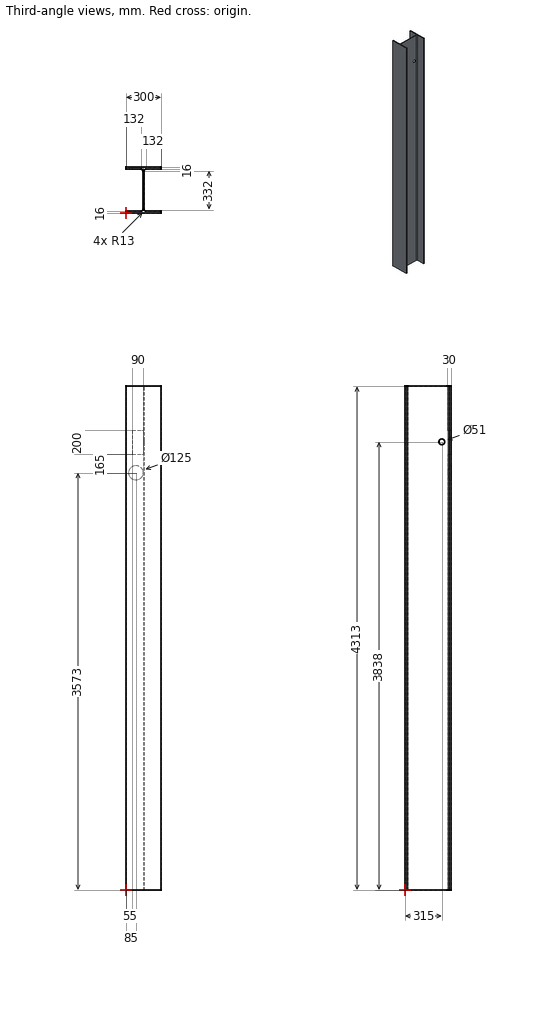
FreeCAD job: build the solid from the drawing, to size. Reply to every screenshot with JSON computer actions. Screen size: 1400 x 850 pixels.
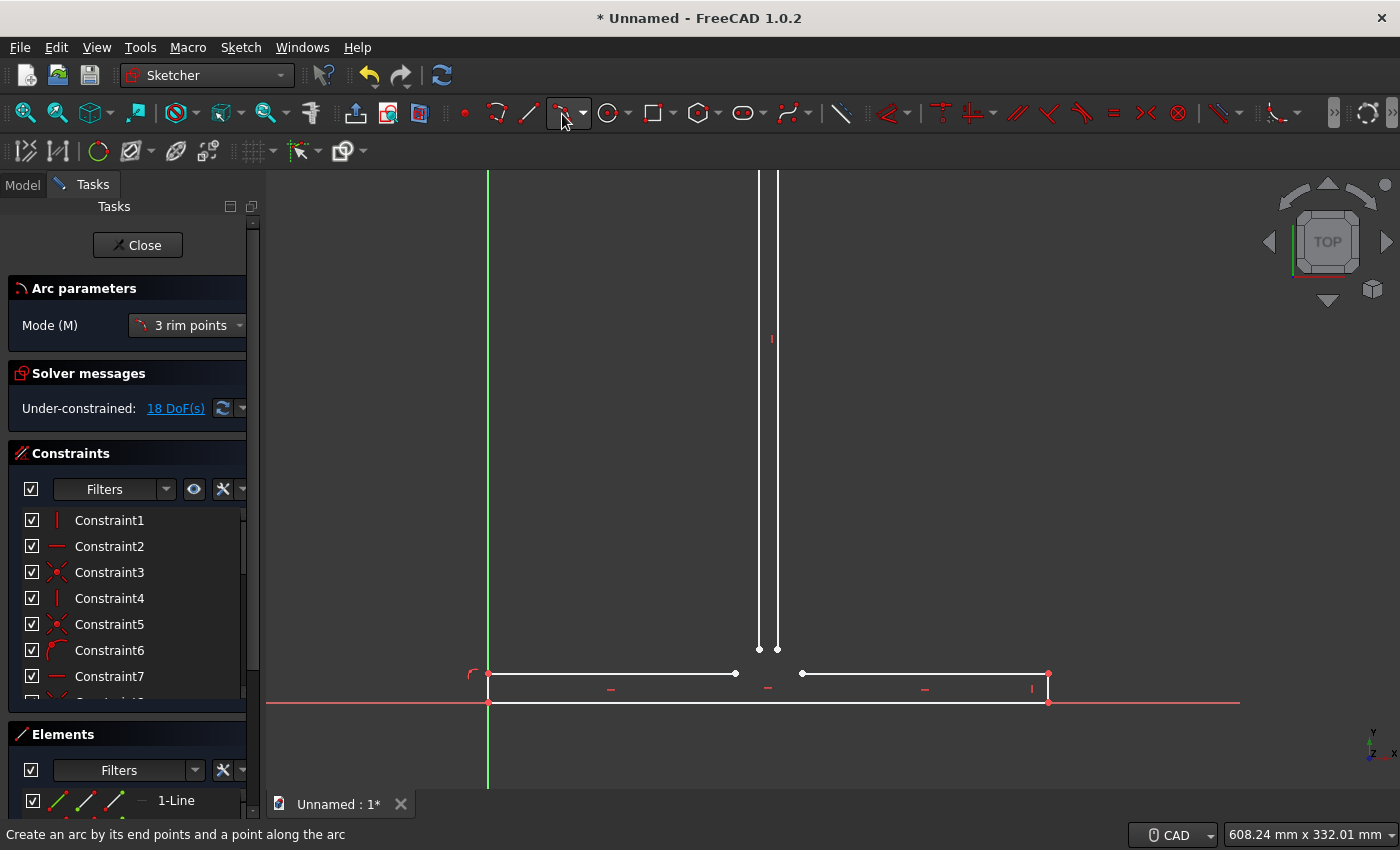
{"action": "scroll", "coordinate": [760, 650], "scroll_direction": "down", "scroll_amount": 3}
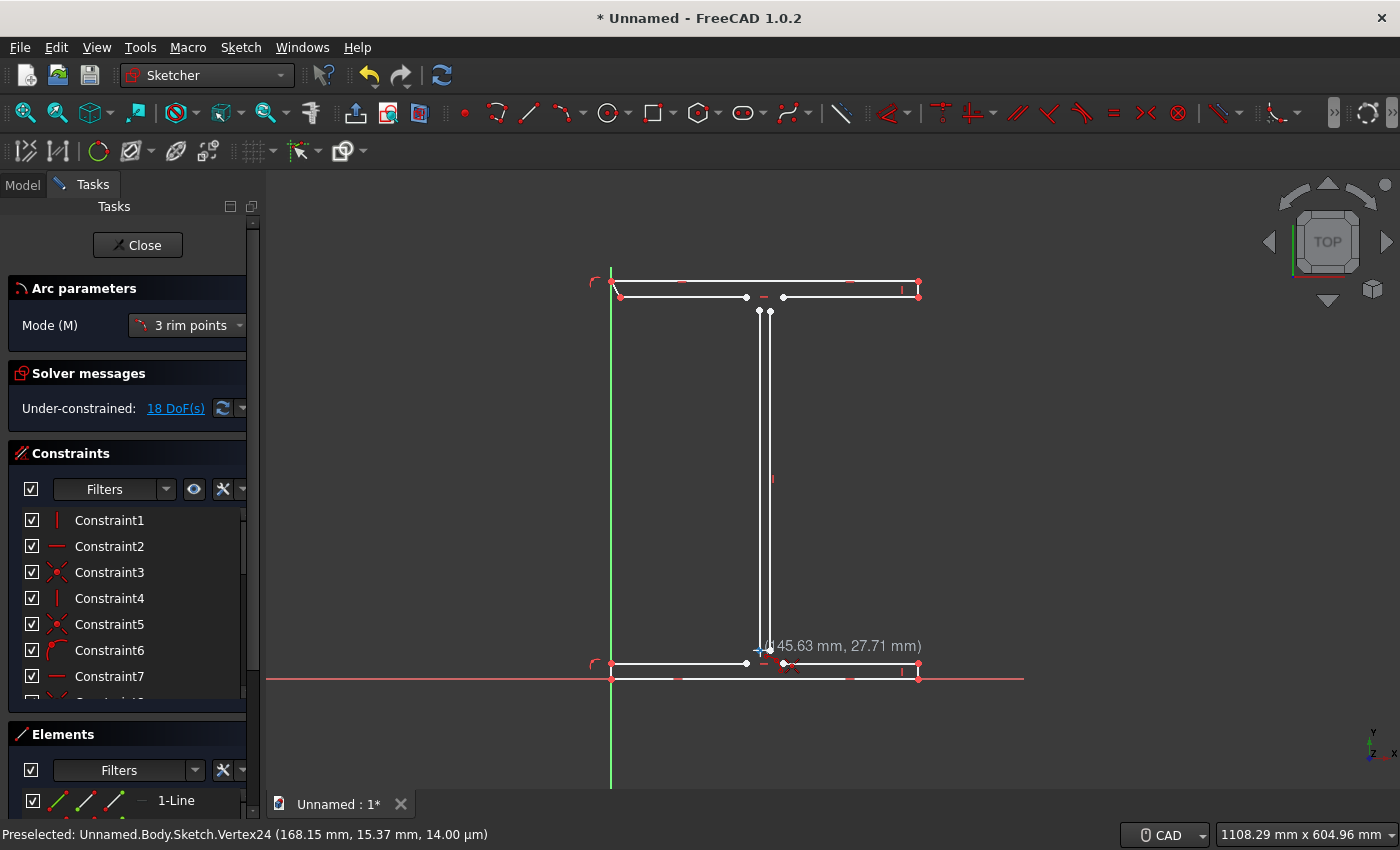
{"action": "scroll", "coordinate": [770, 310], "scroll_direction": "up", "scroll_amount": 3}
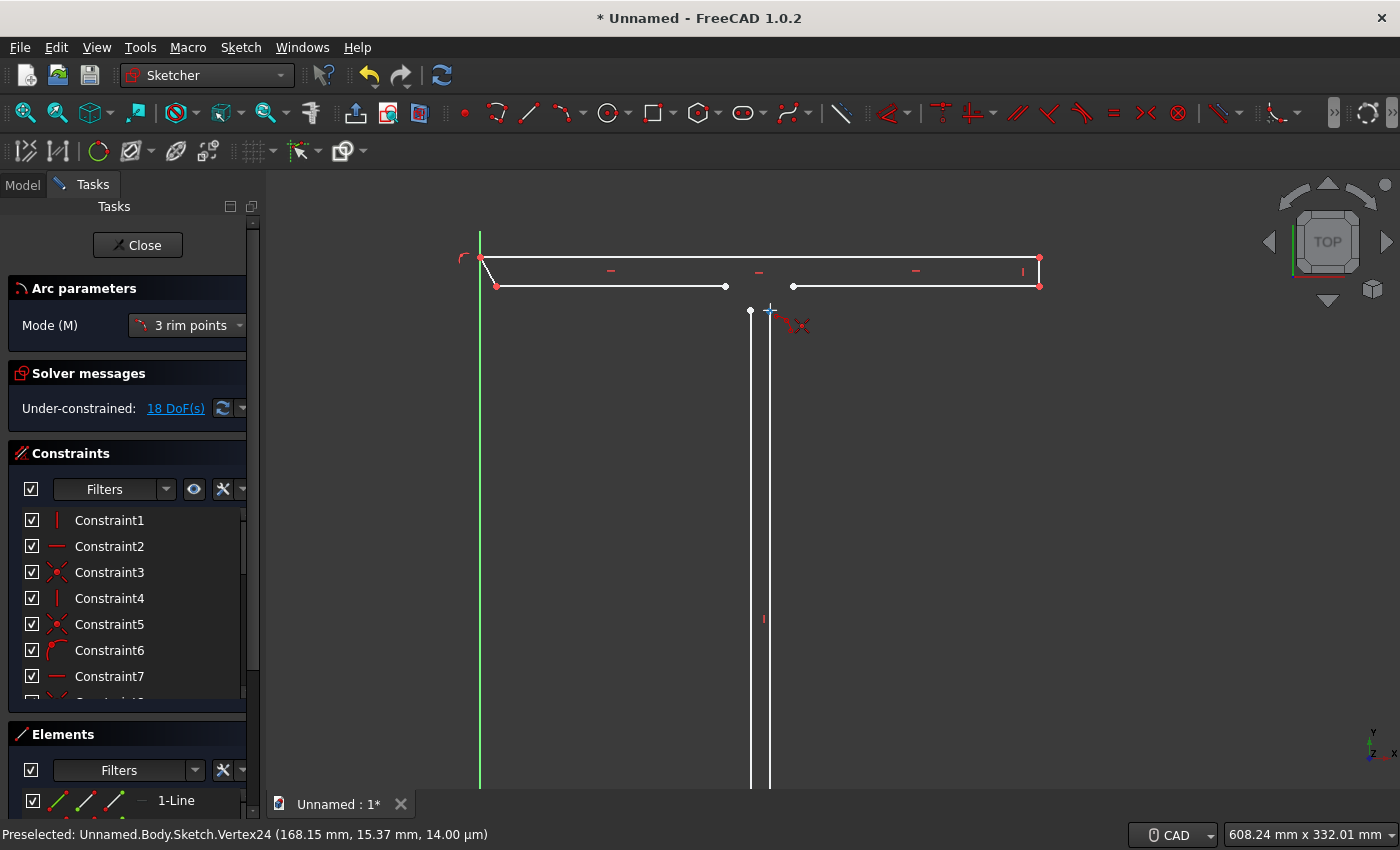
{"action": "left_click", "coordinate": [770, 312]}
{"action": "left_click", "coordinate": [793, 286]}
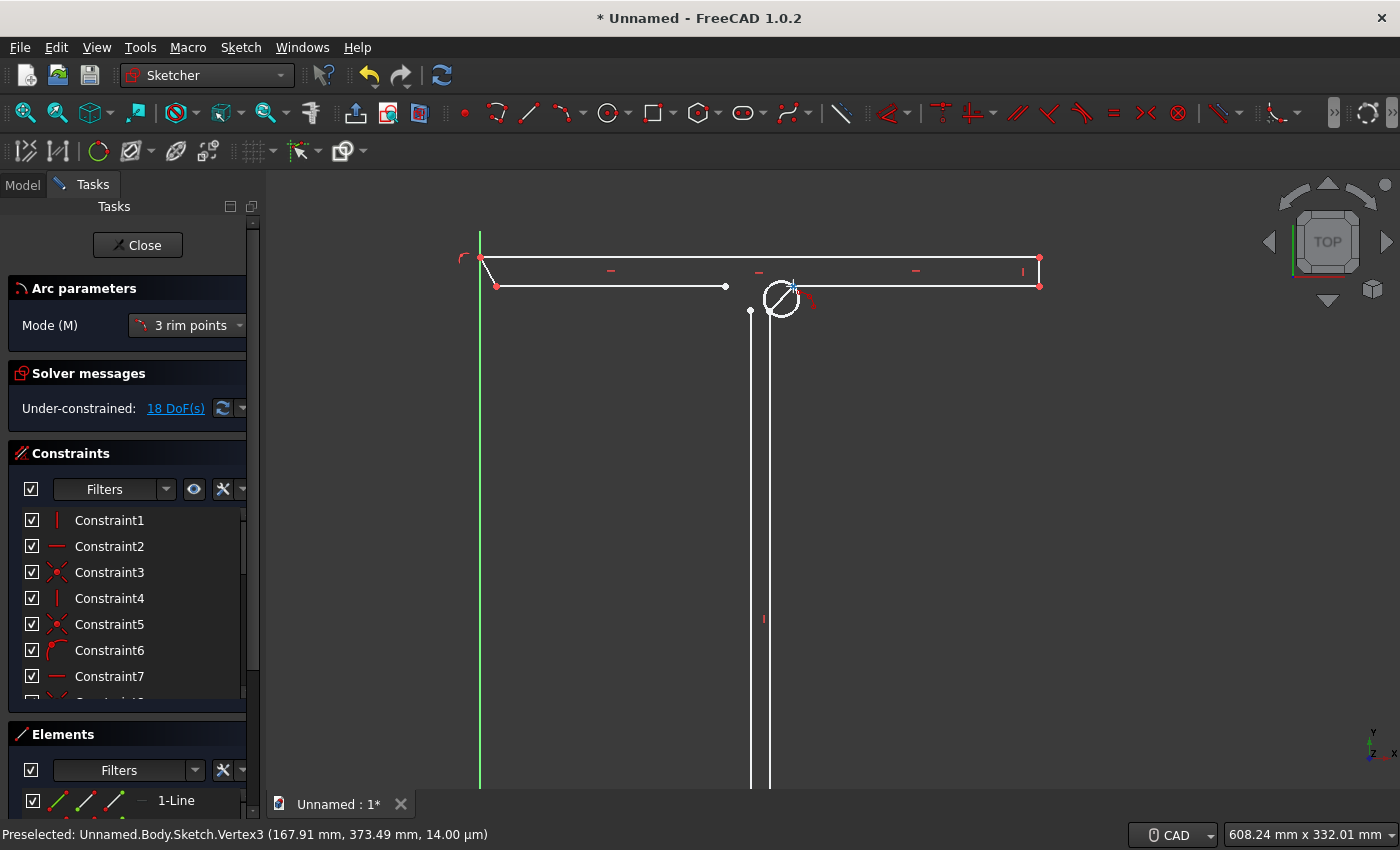
{"action": "scroll", "coordinate": [776, 292], "scroll_direction": "up", "scroll_amount": 5}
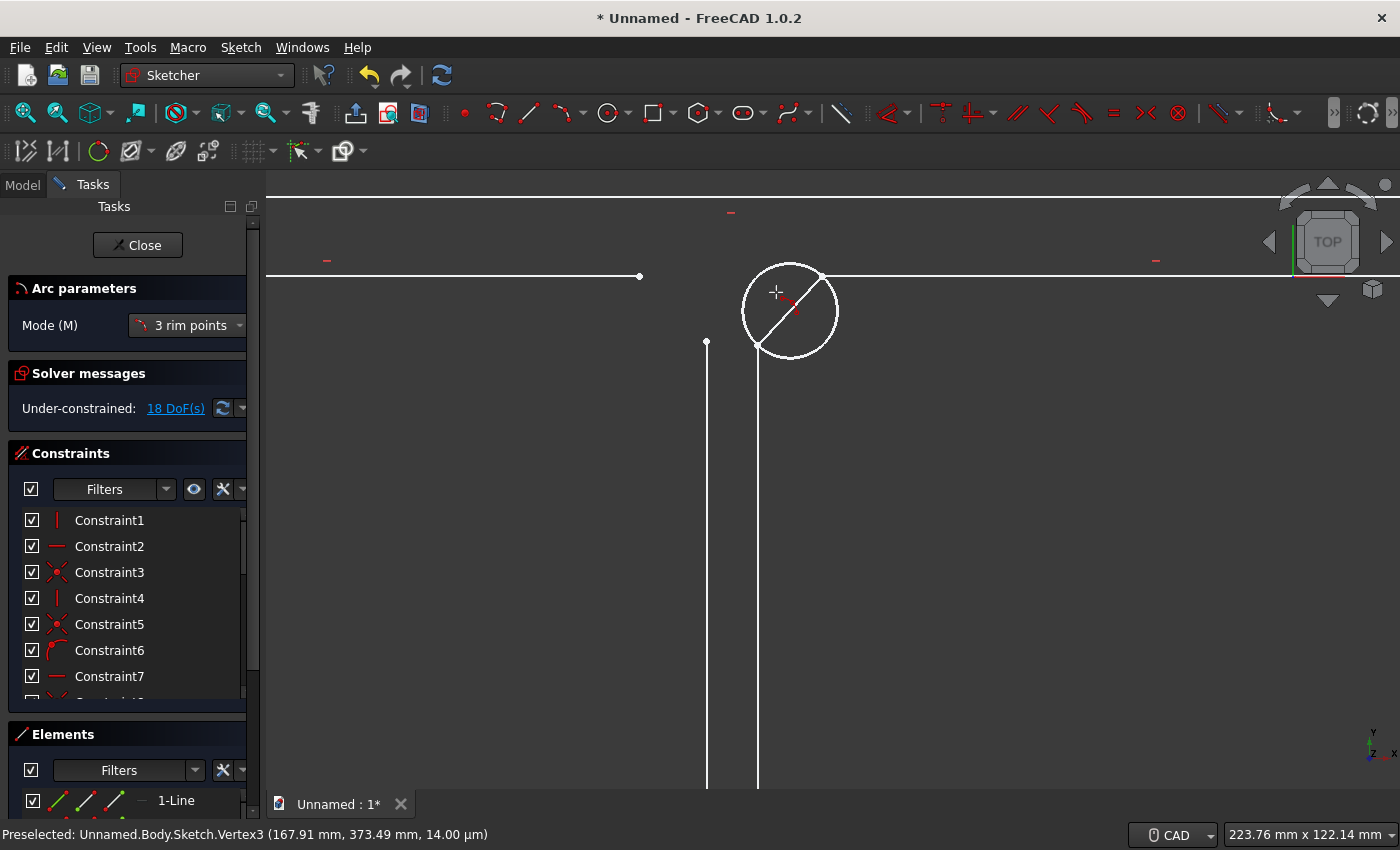
{"action": "left_click", "coordinate": [776, 293]}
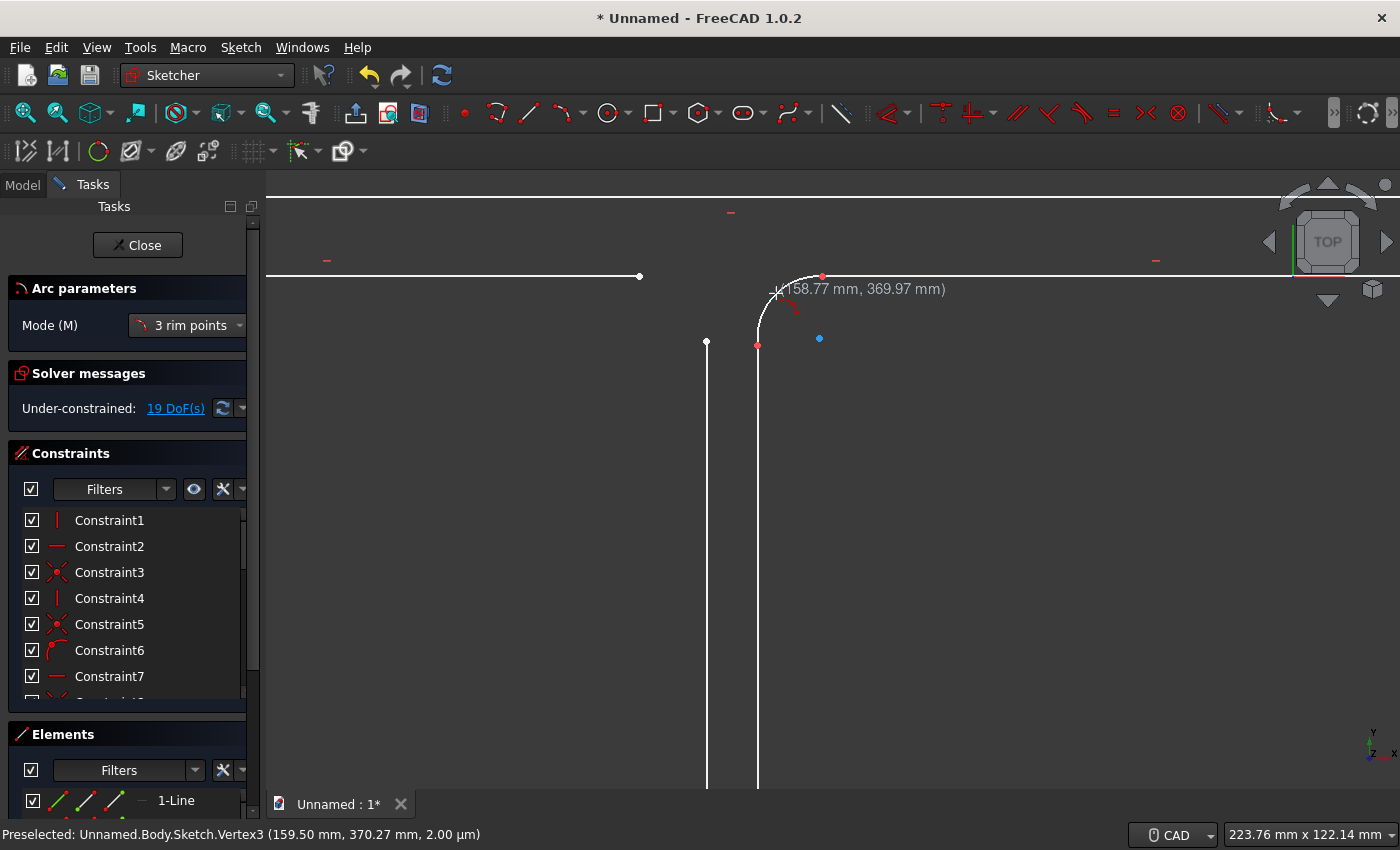
{"action": "scroll", "coordinate": [773, 302], "scroll_direction": "down", "scroll_amount": 8}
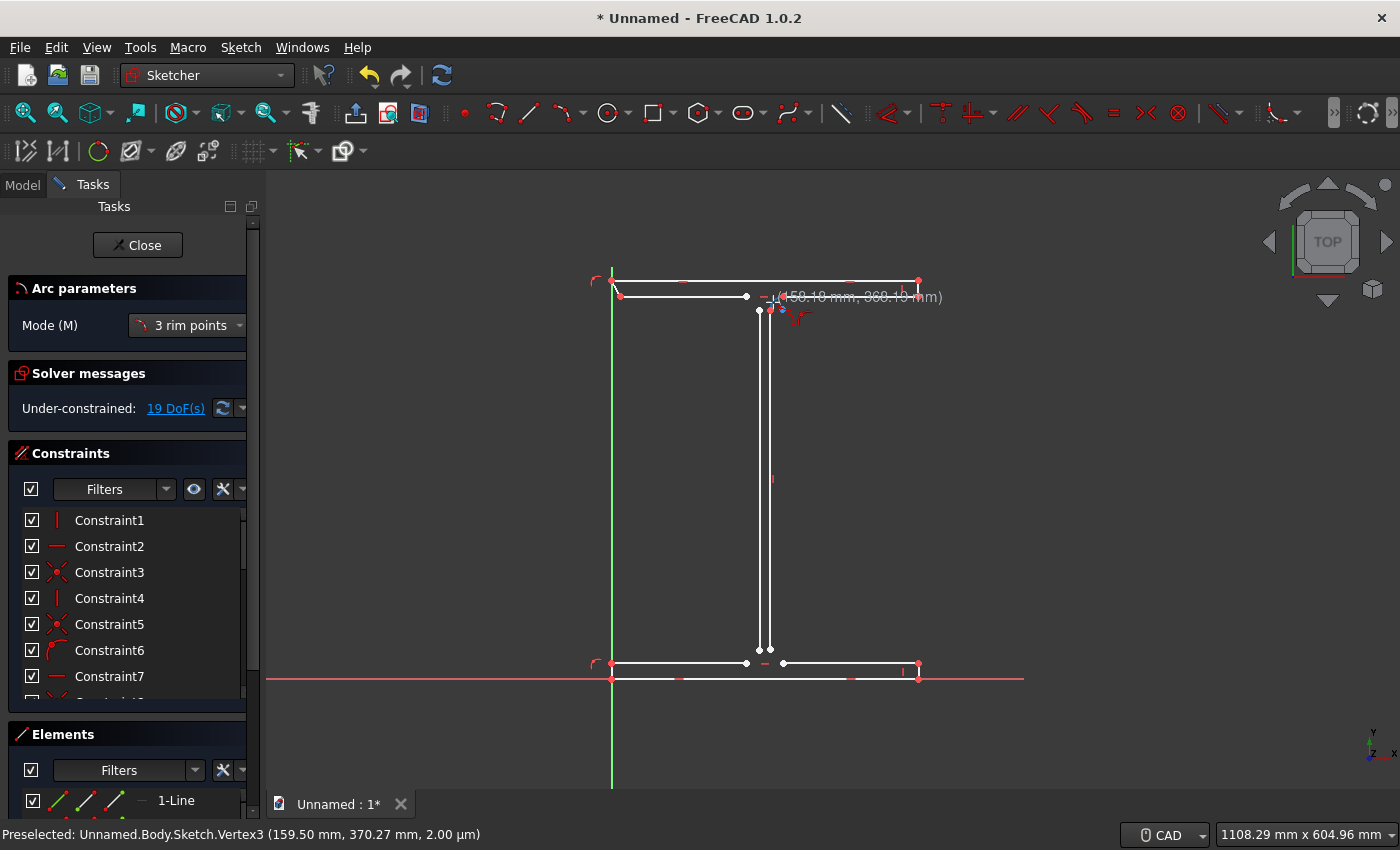
{"action": "left_click", "coordinate": [746, 297]}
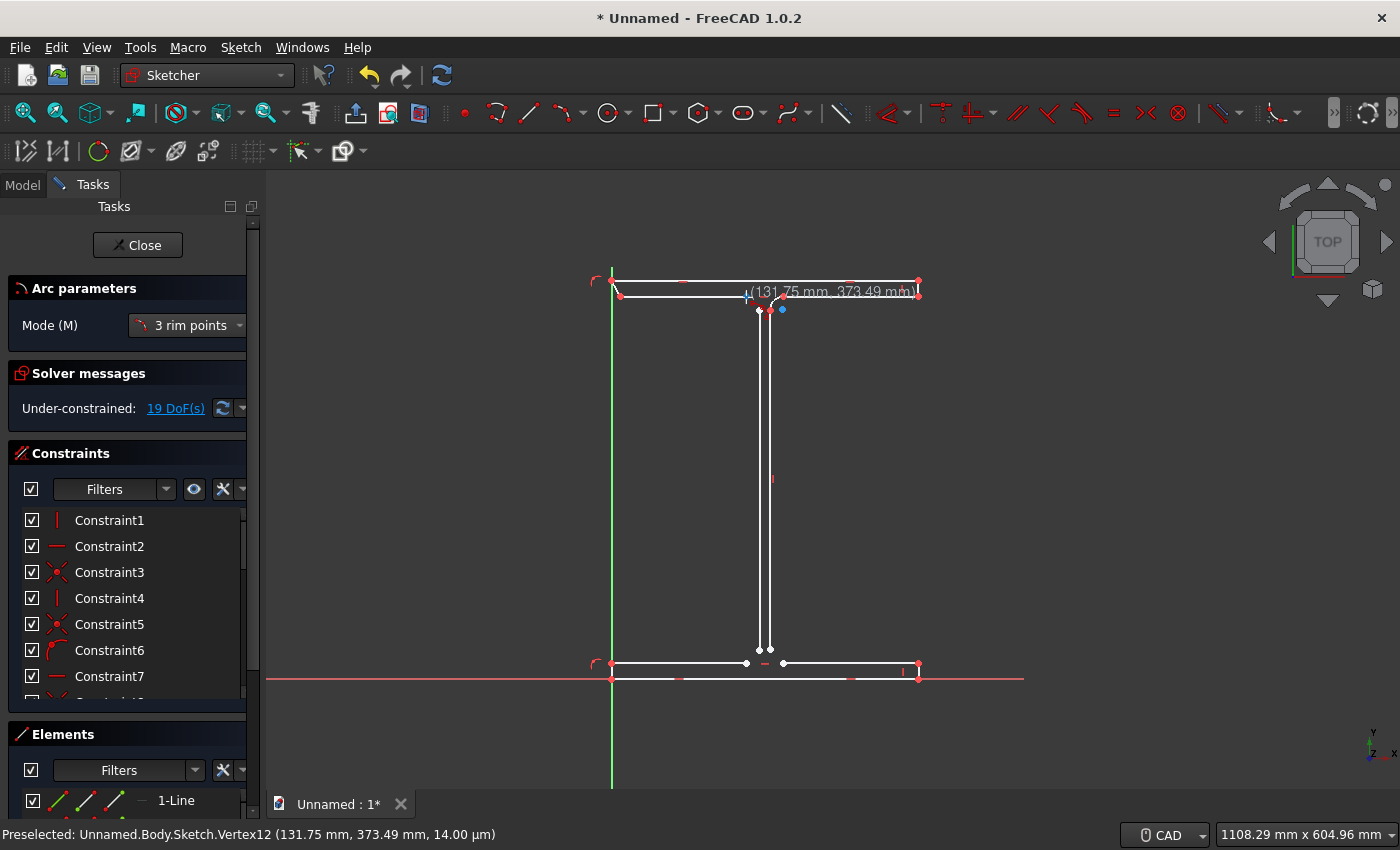
{"action": "scroll", "coordinate": [760, 310], "scroll_direction": "up", "scroll_amount": 3}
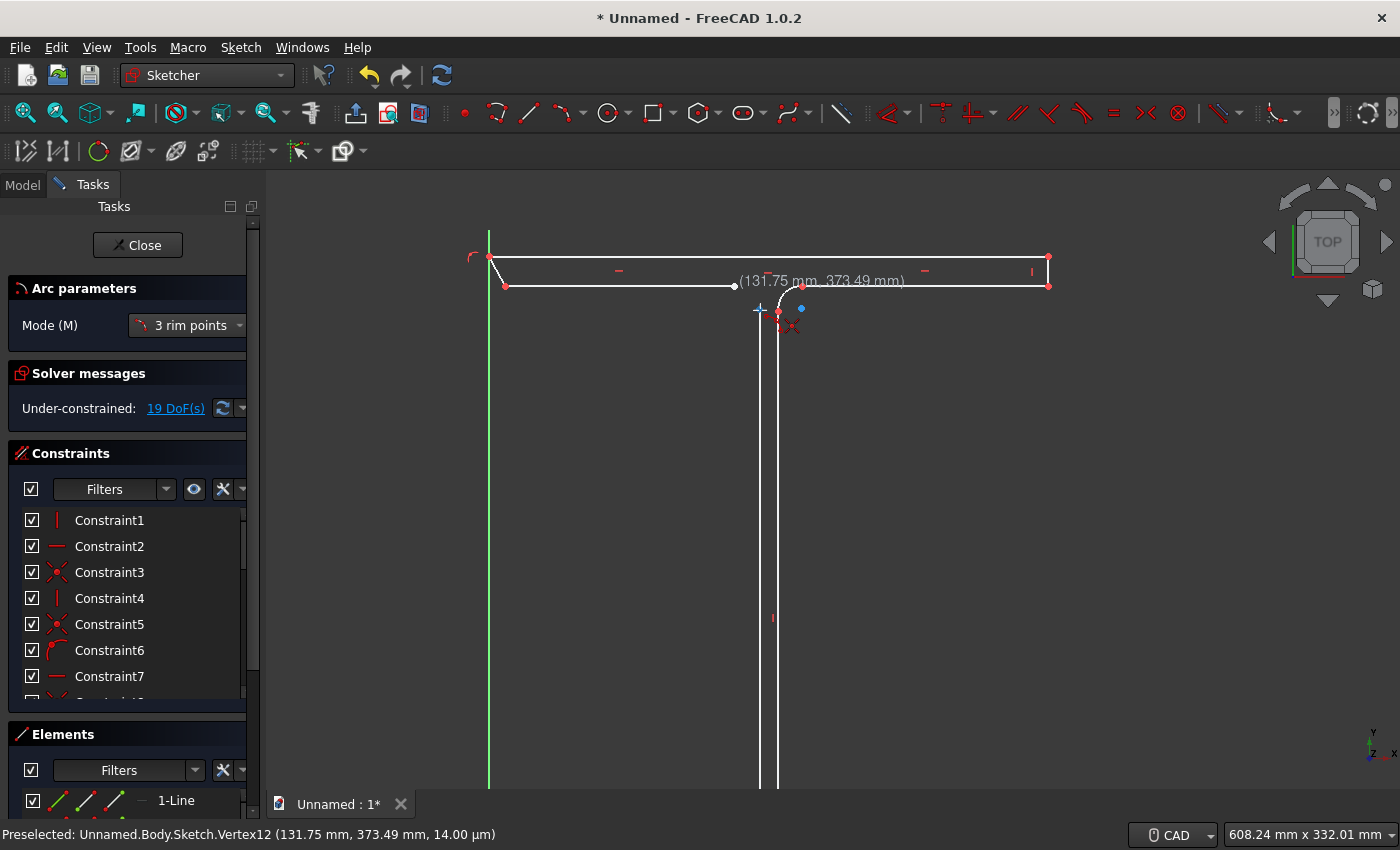
{"action": "left_click", "coordinate": [760, 310]}